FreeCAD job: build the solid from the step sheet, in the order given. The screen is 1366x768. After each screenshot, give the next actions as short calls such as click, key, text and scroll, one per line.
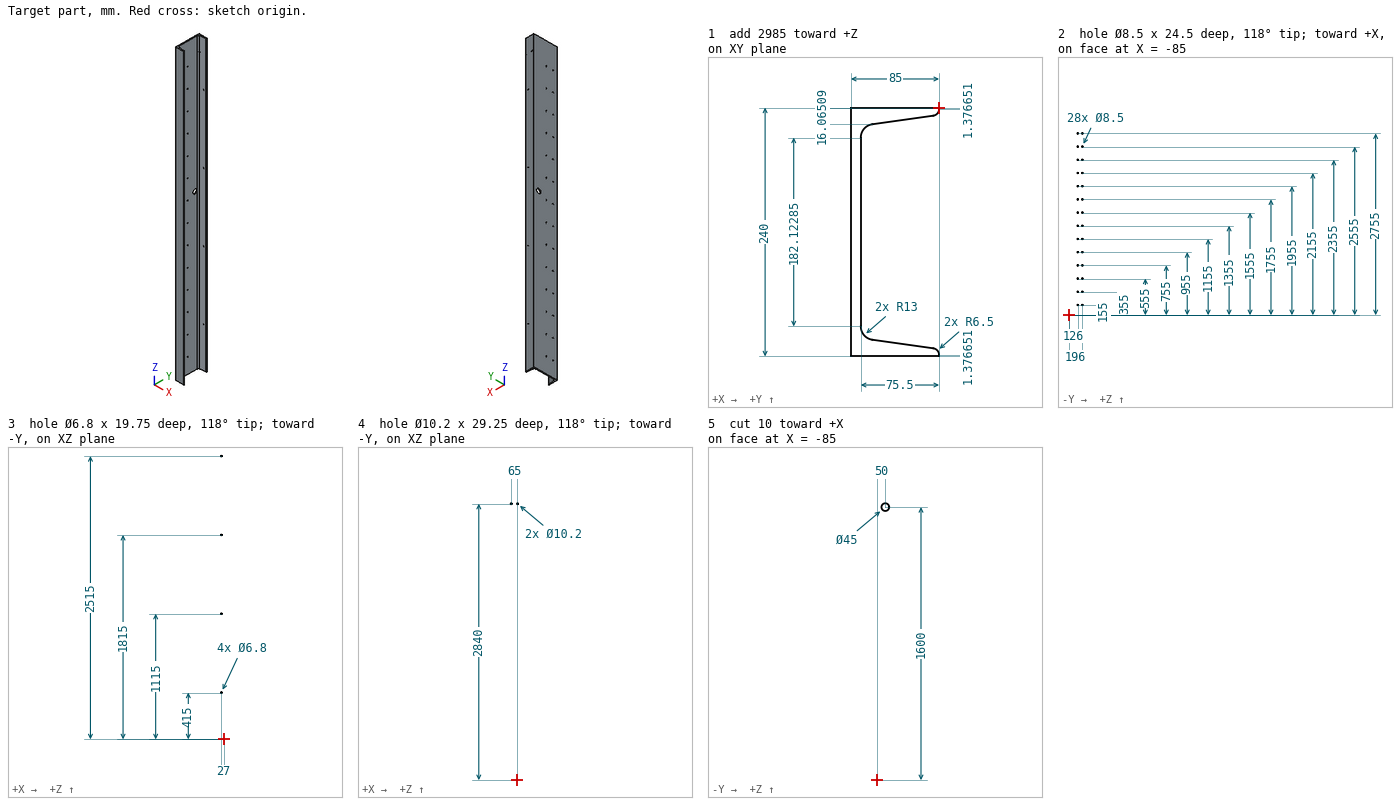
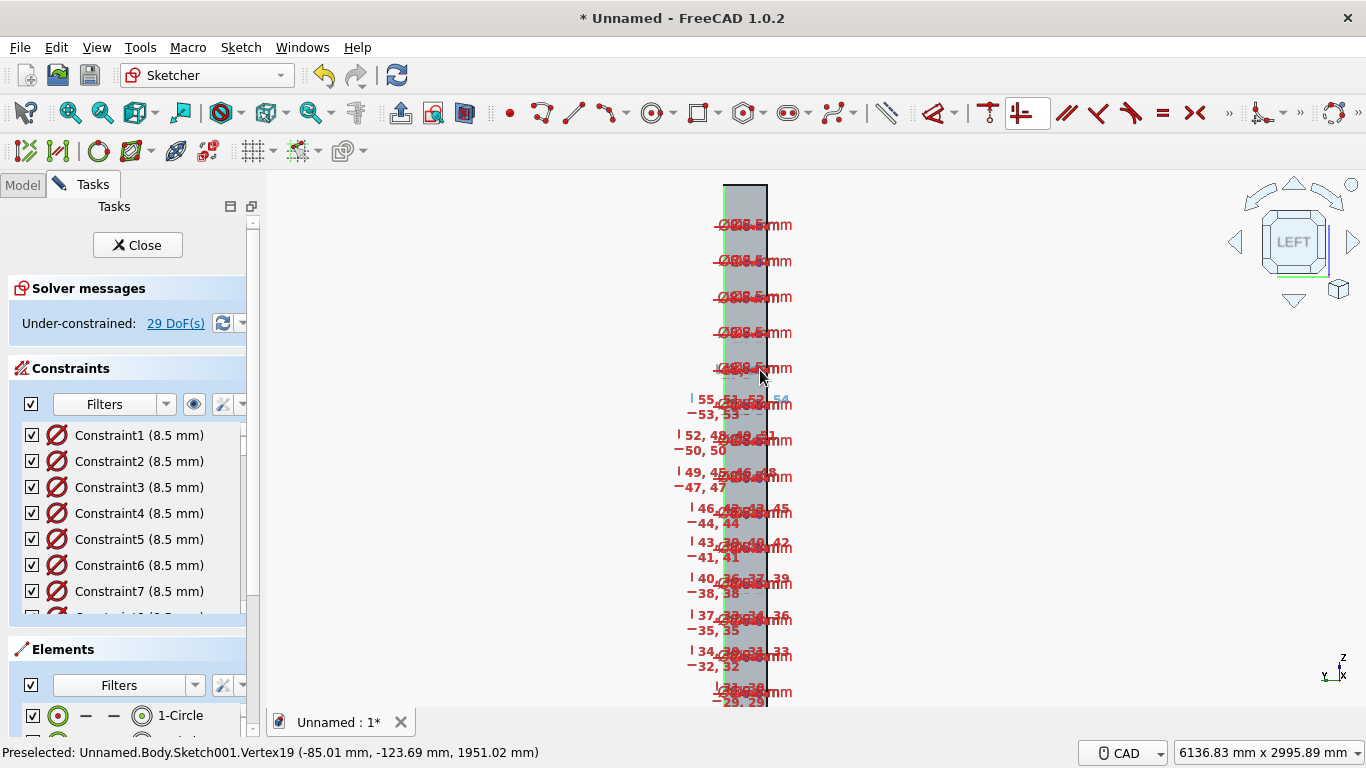
scroll(759, 370, up, 4)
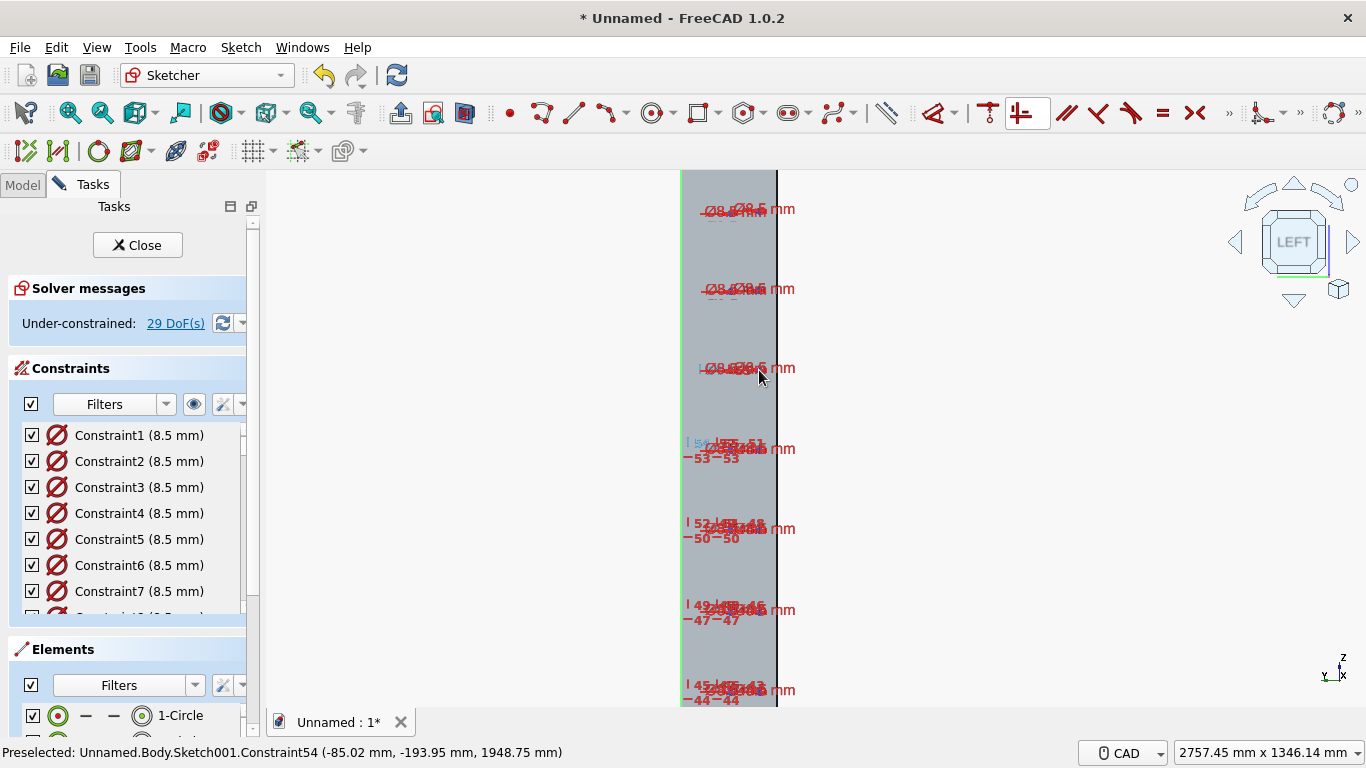
click(759, 370)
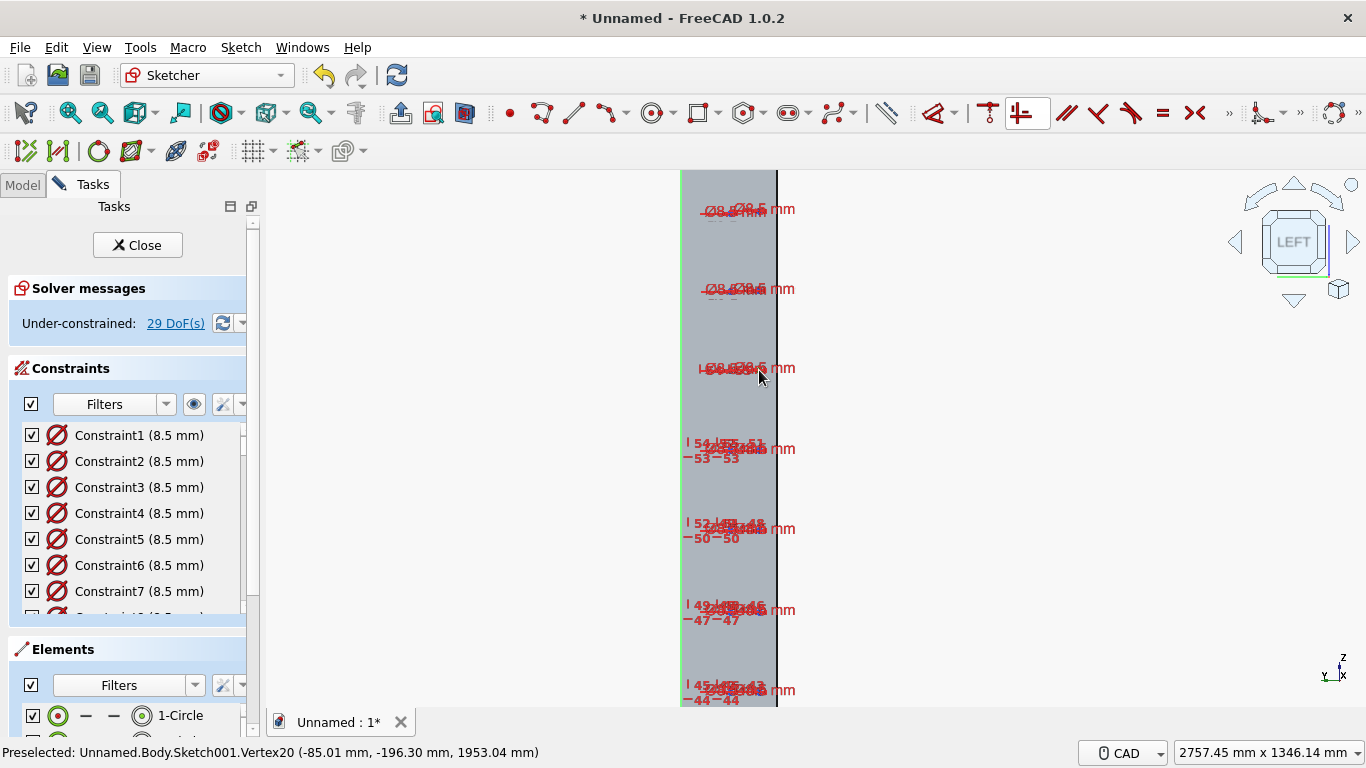
key(h)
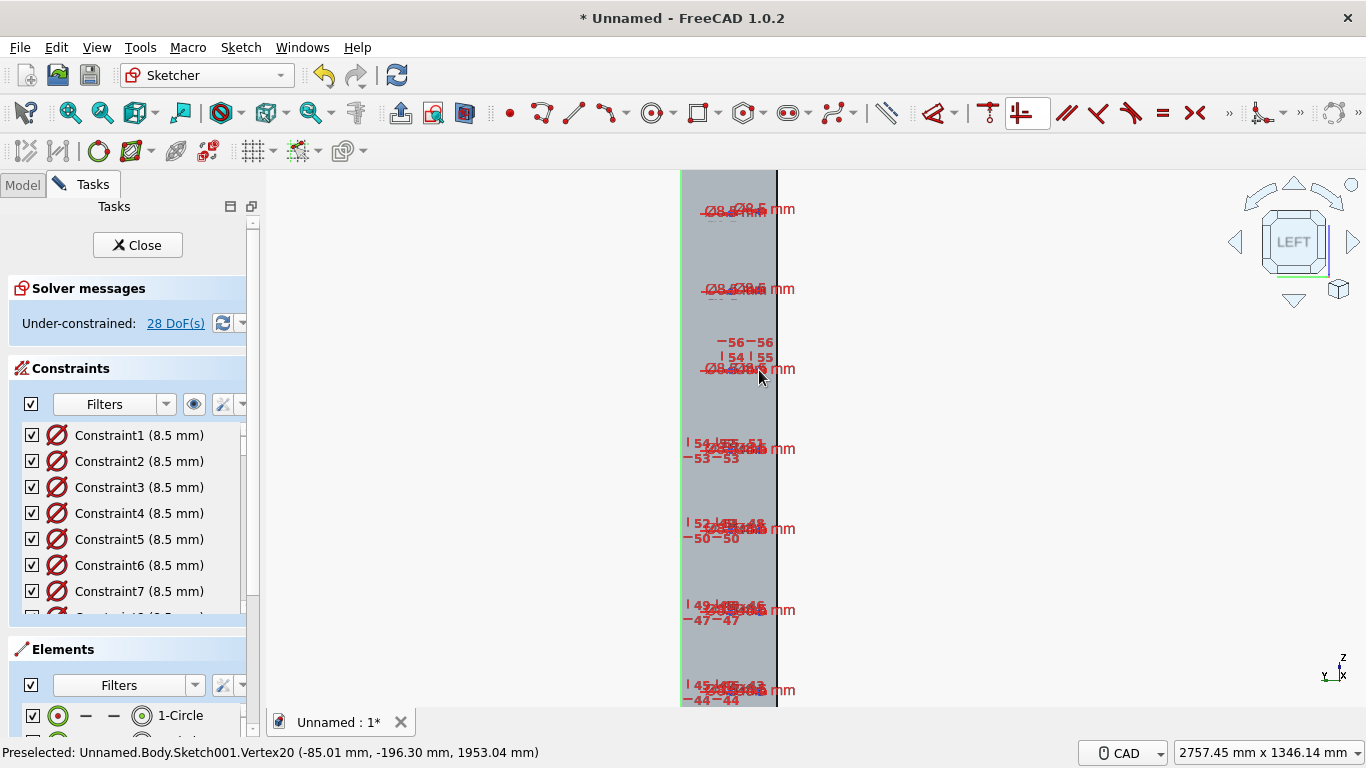
click(759, 371)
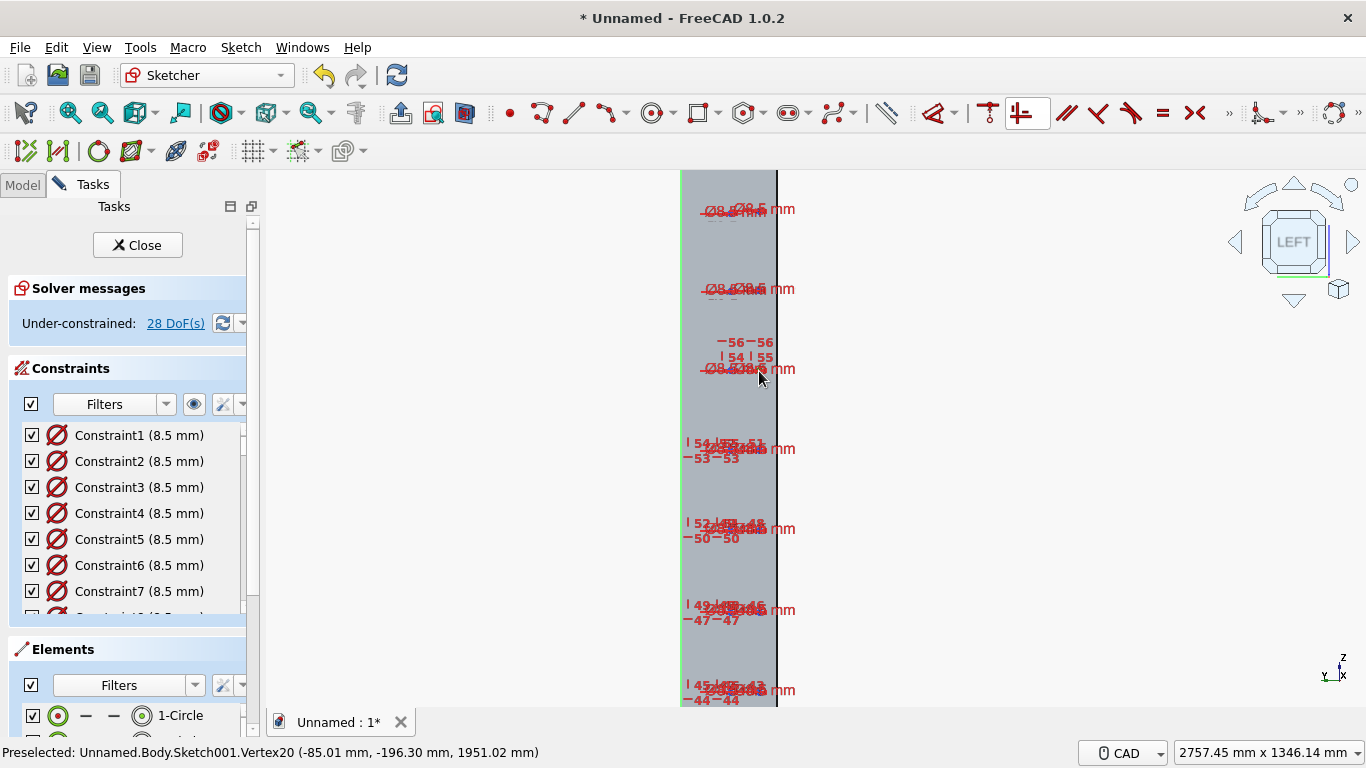
click(759, 291)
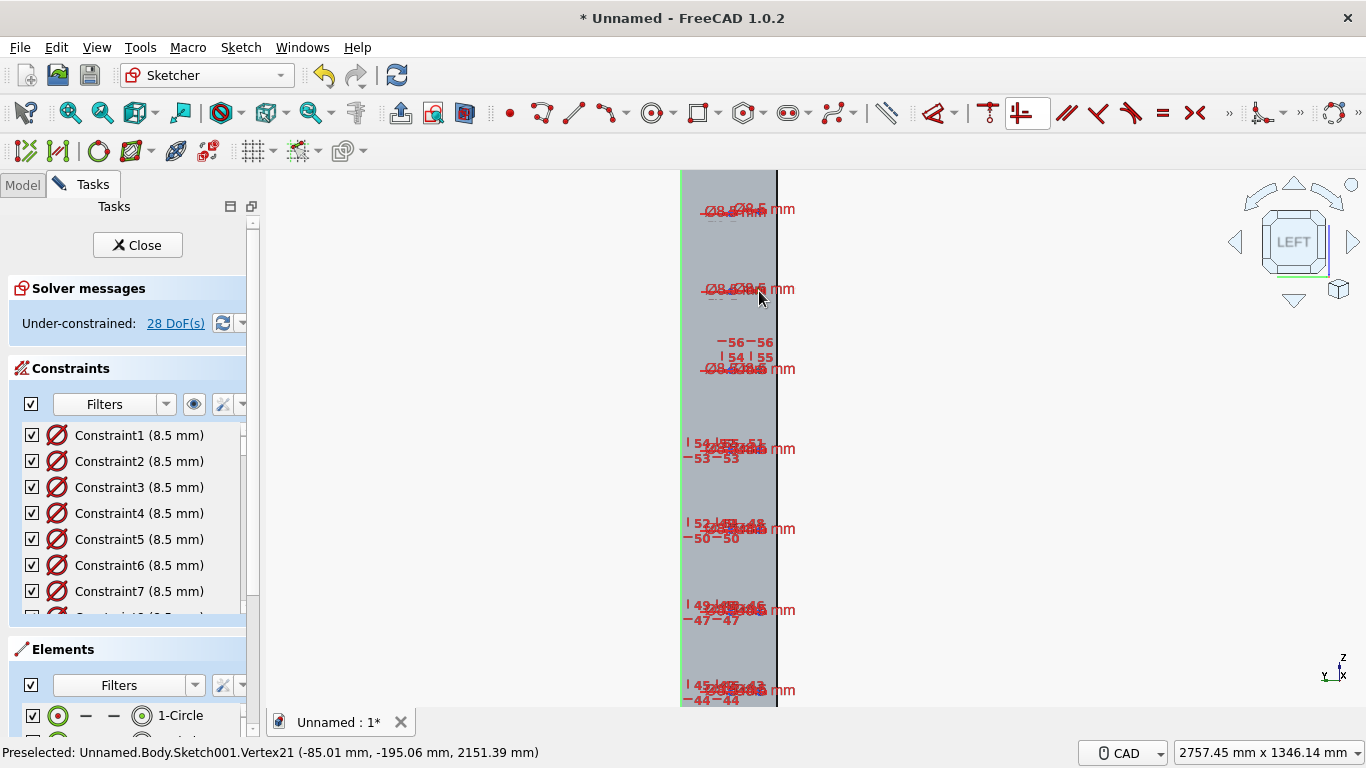
key(v)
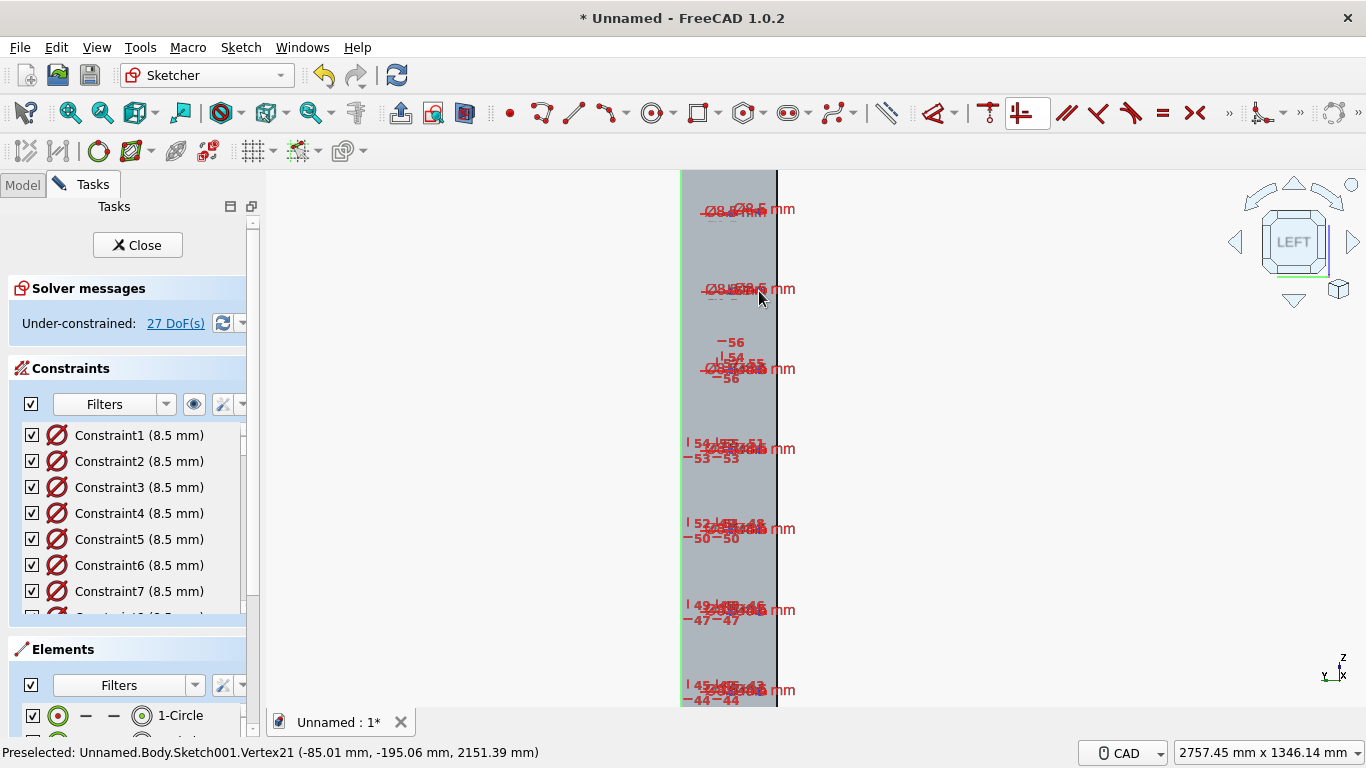
click(730, 371)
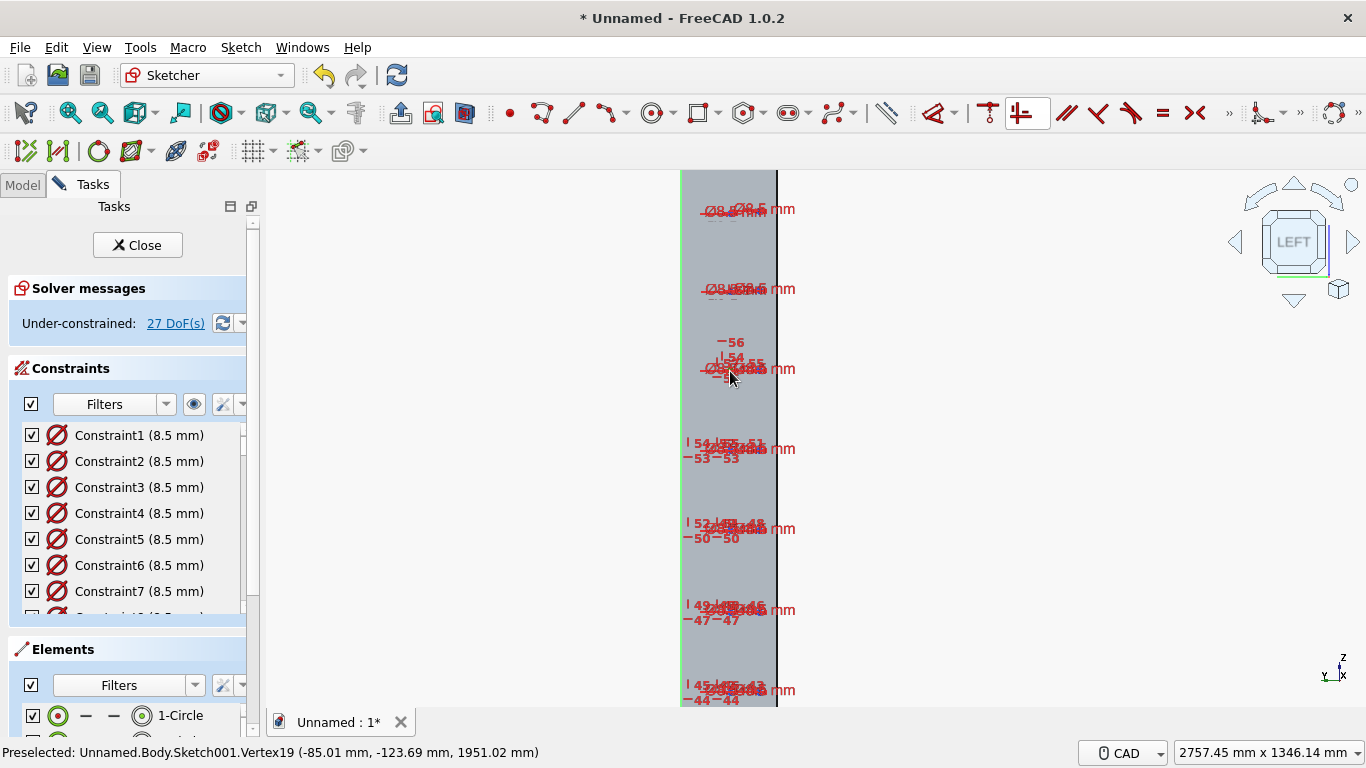
scroll(731, 292, up, 4)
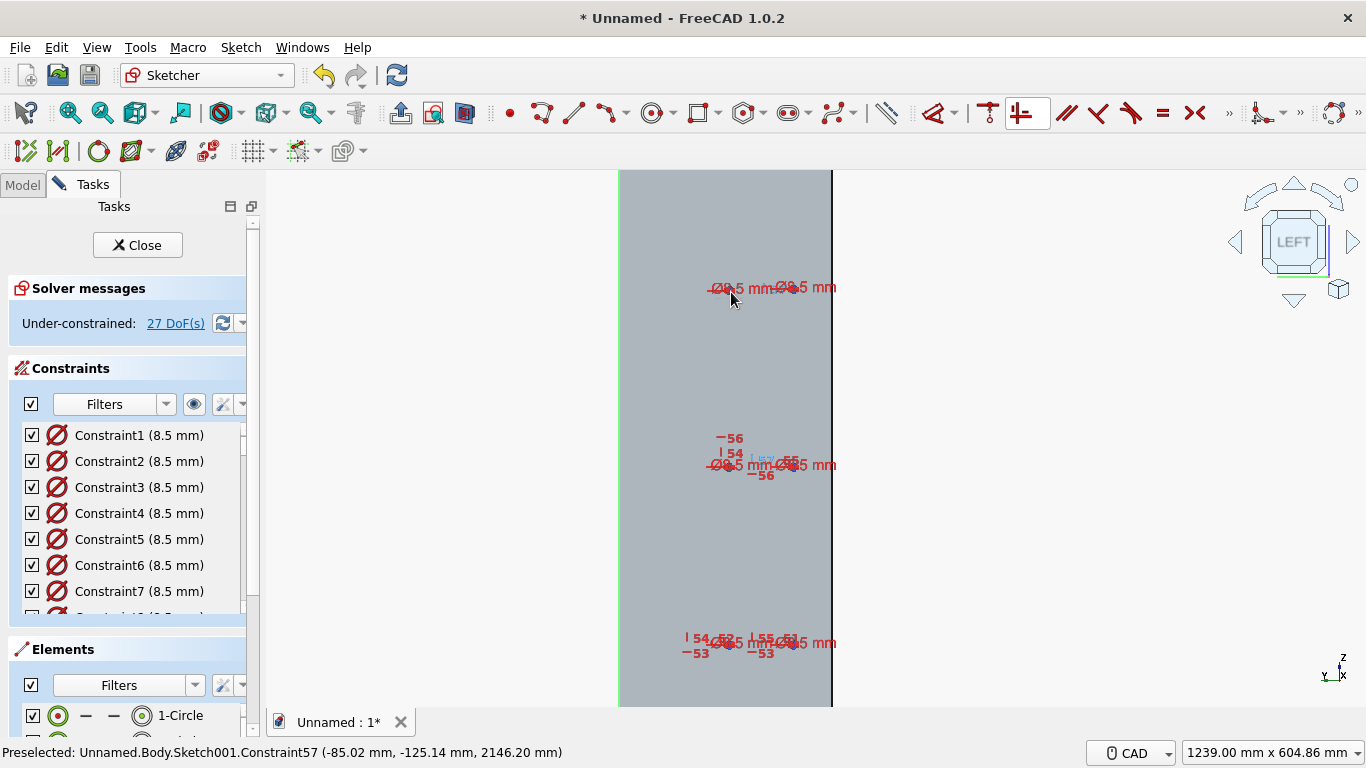
click(730, 291)